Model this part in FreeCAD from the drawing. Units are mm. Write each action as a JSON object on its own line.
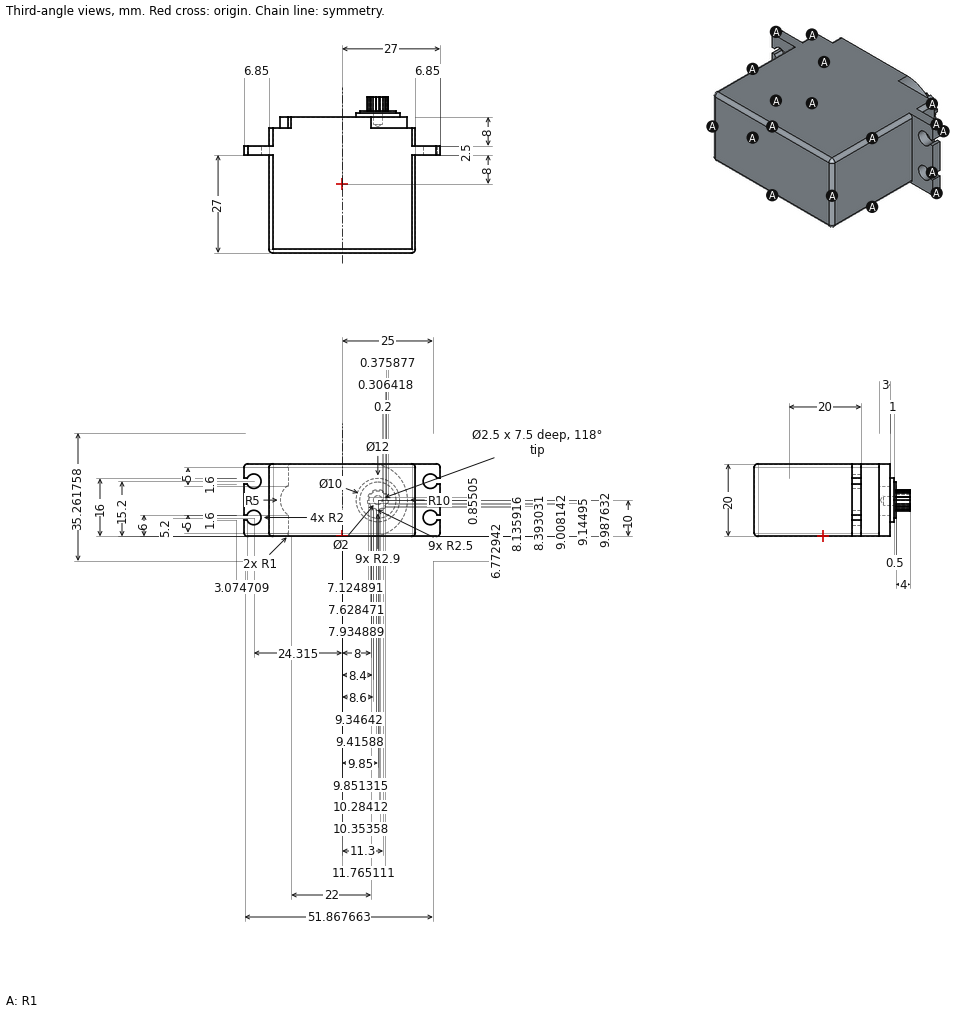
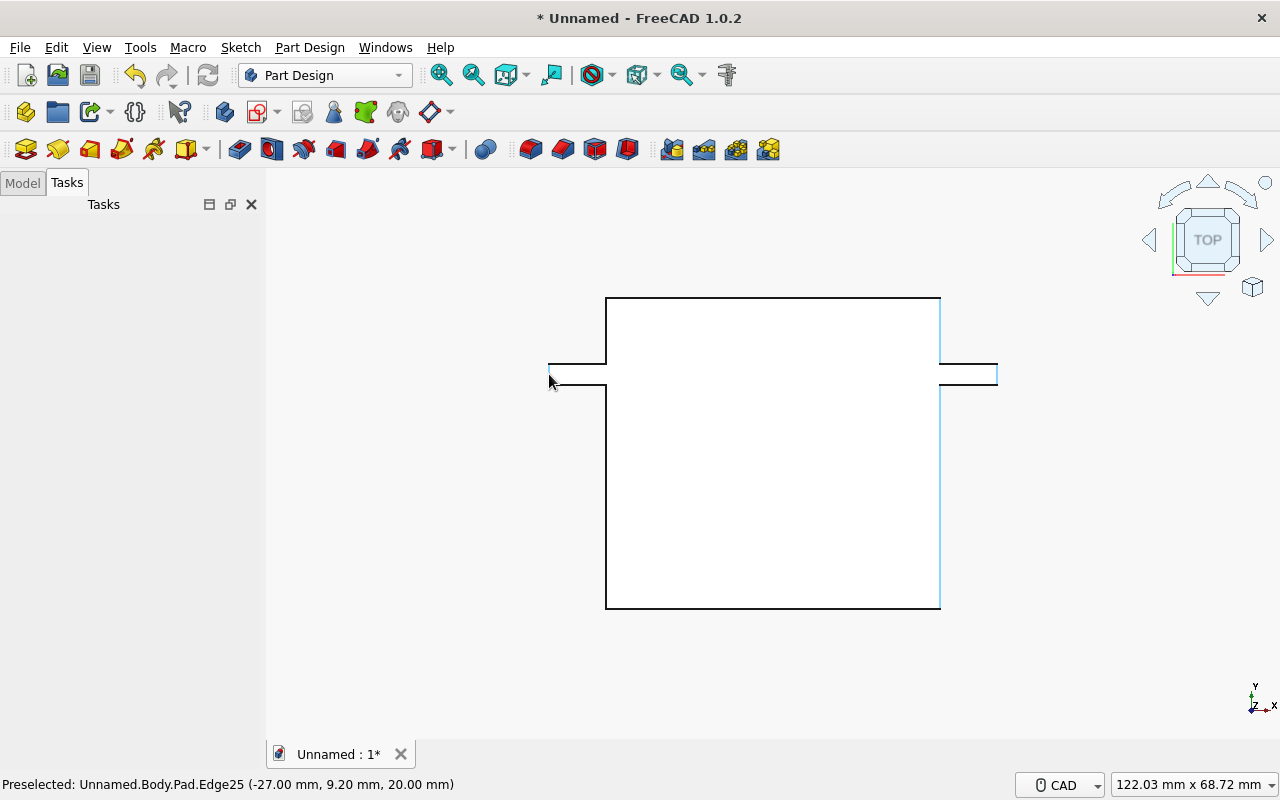
{"action": "left_click", "coordinate": [606, 496], "text": "ctrl"}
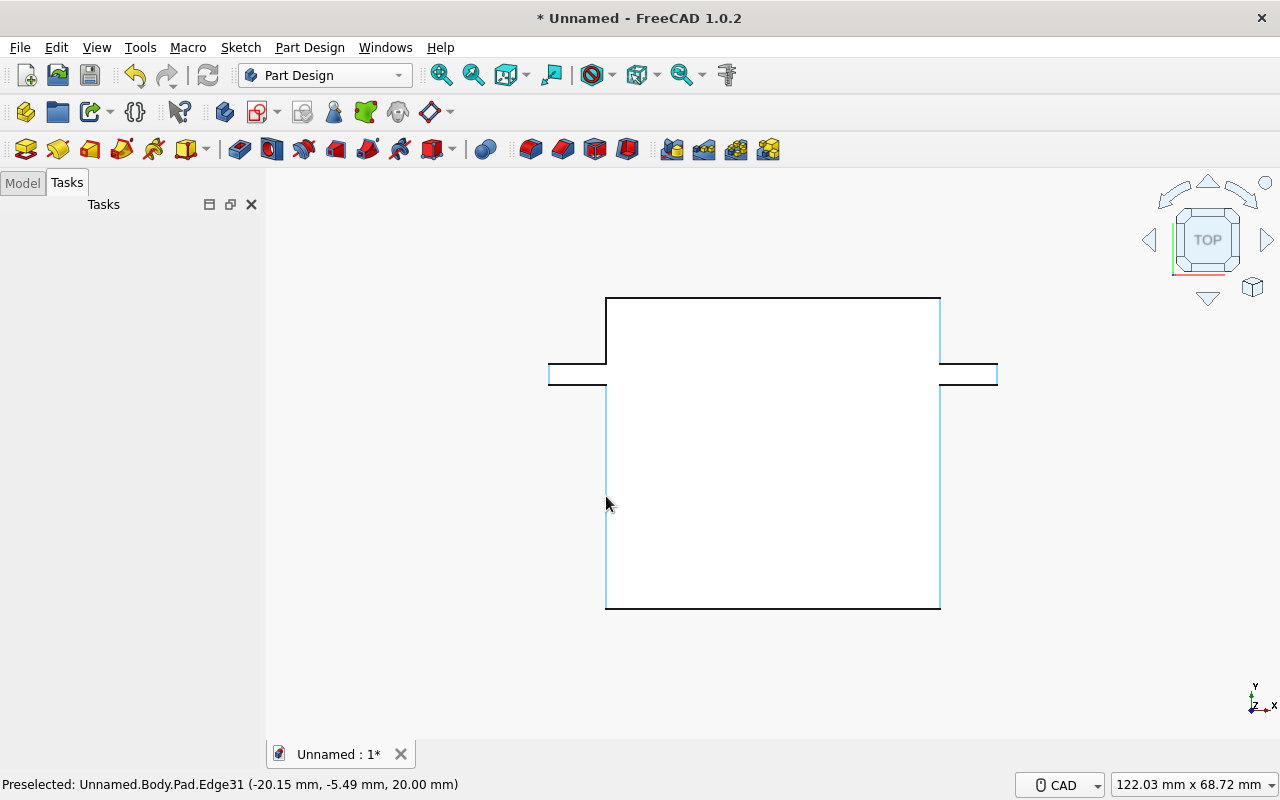
{"action": "left_click", "coordinate": [606, 330], "text": "ctrl"}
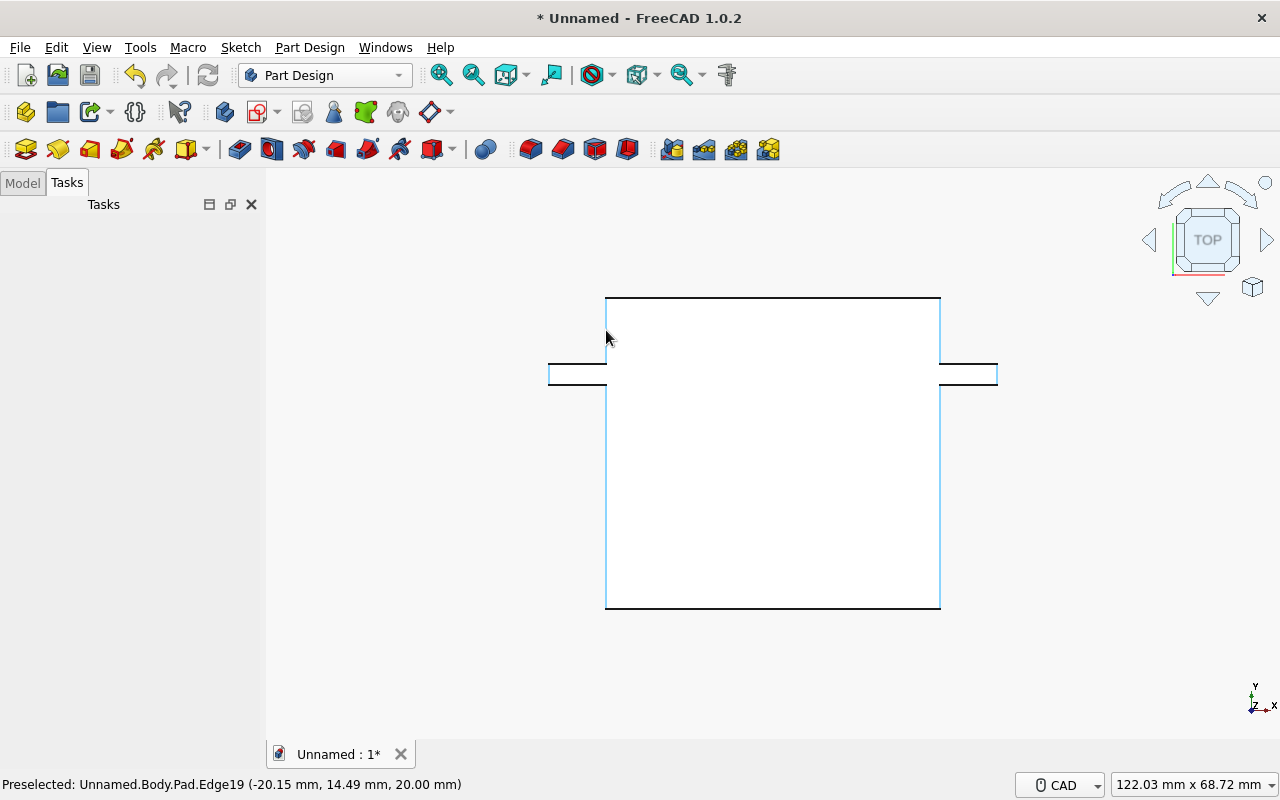
{"action": "key", "text": "1"}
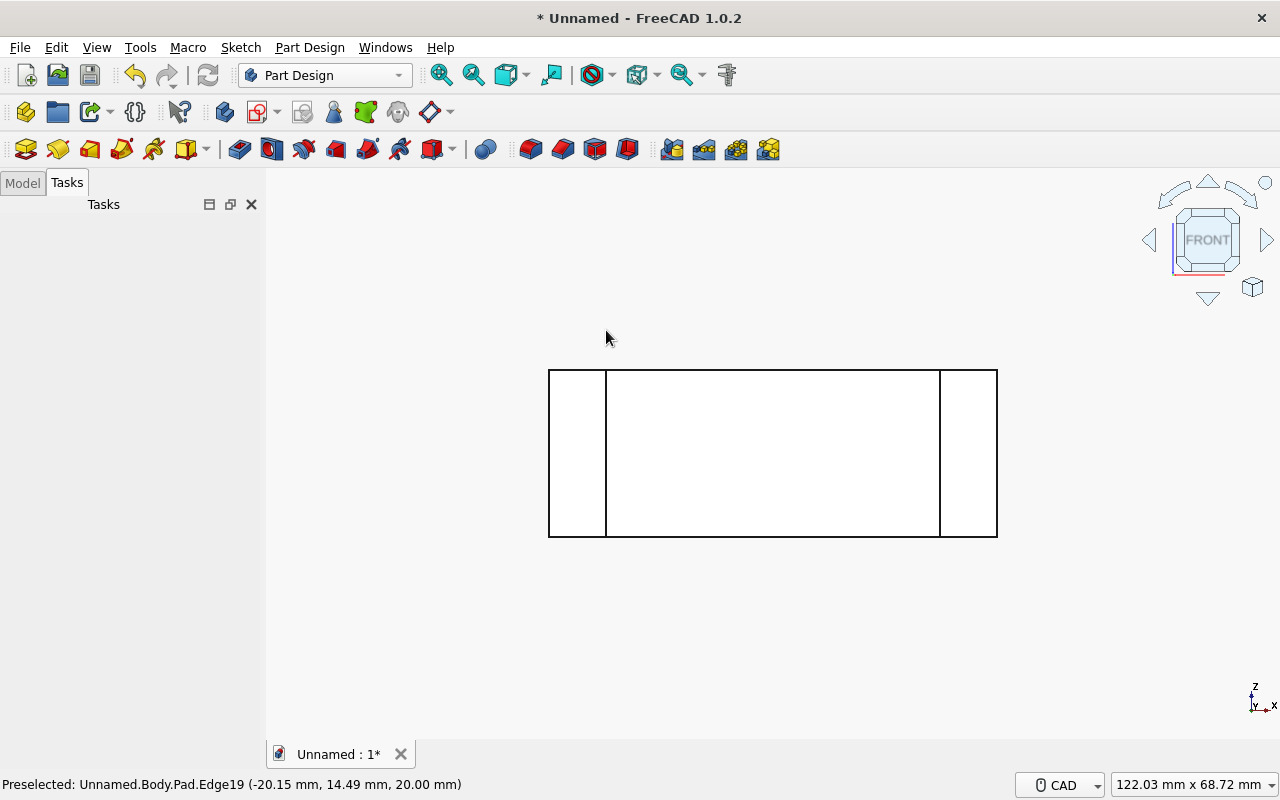
{"action": "key", "text": "v f"}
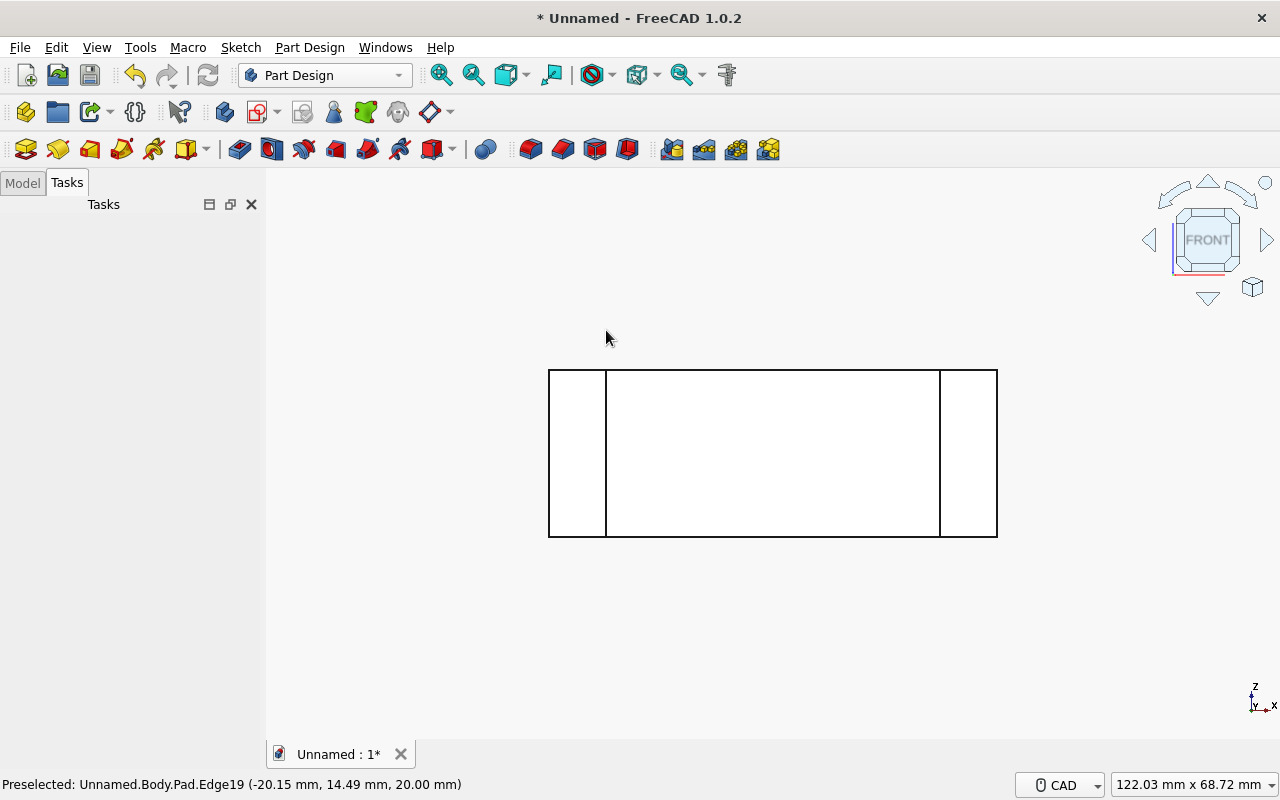
{"action": "key", "text": "3"}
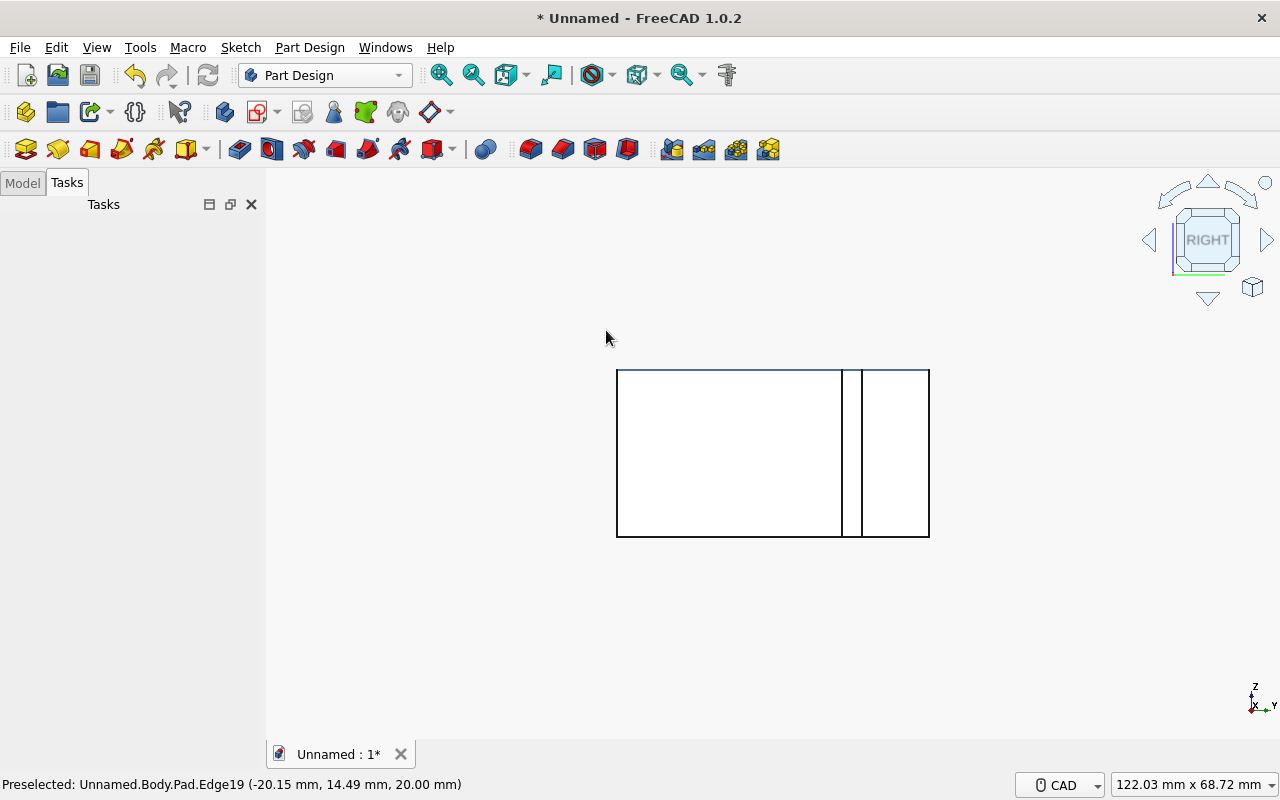
{"action": "key", "text": "v f"}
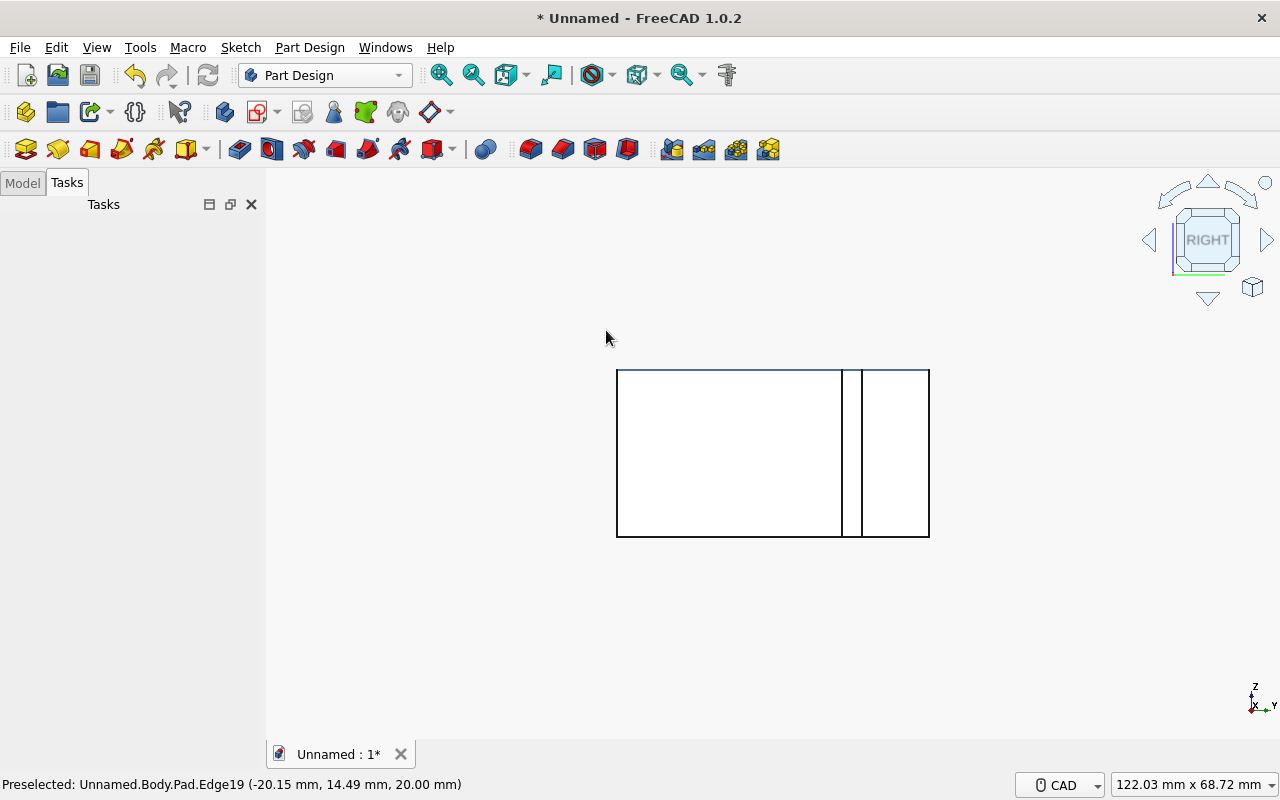
{"action": "left_click", "coordinate": [896, 536], "text": "ctrl"}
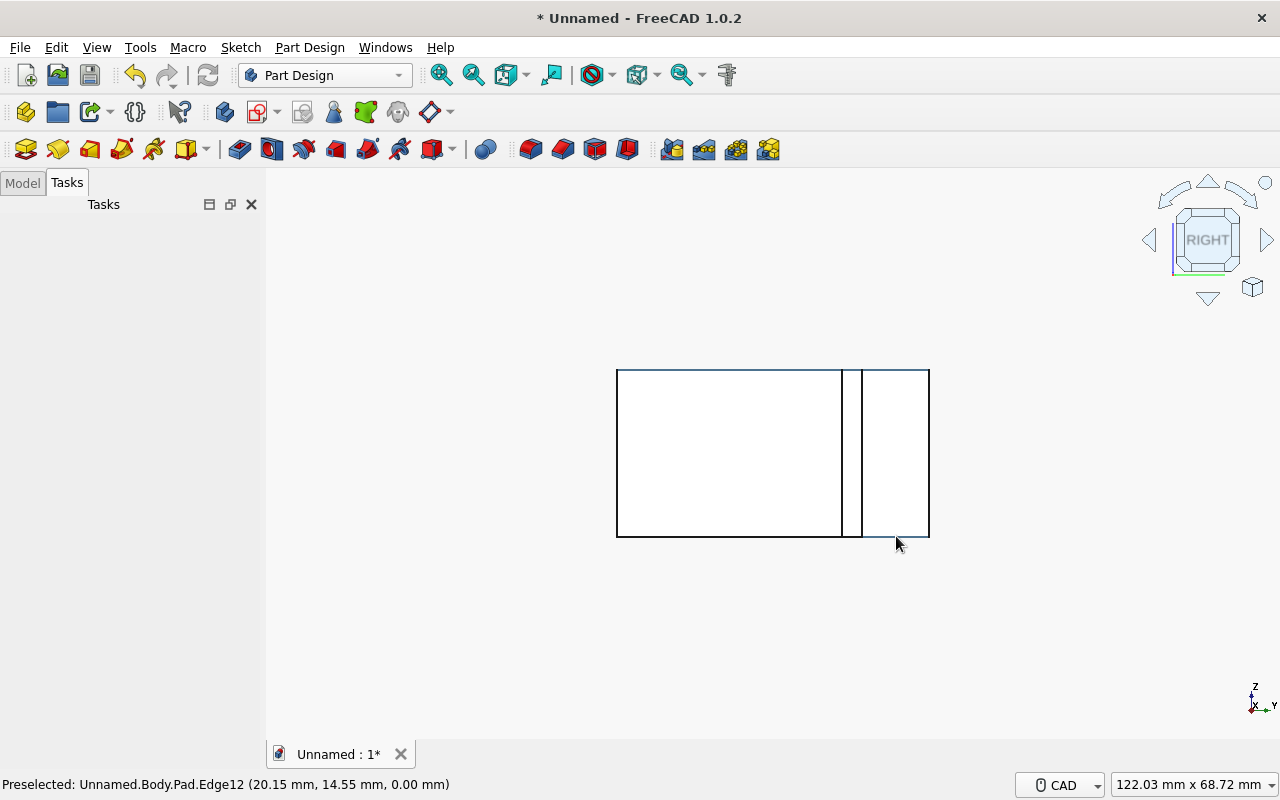
{"action": "left_click", "coordinate": [852, 536], "text": "ctrl"}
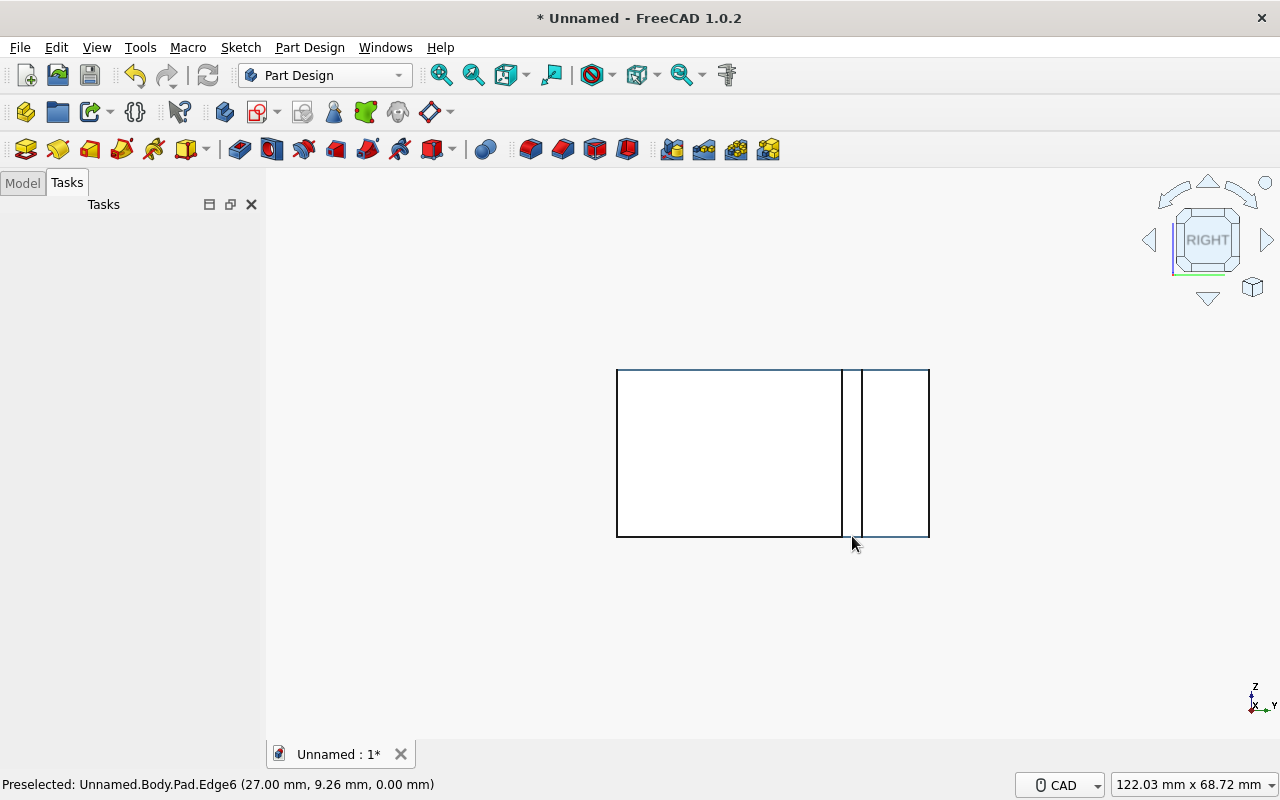
{"action": "left_click", "coordinate": [729, 536], "text": "ctrl"}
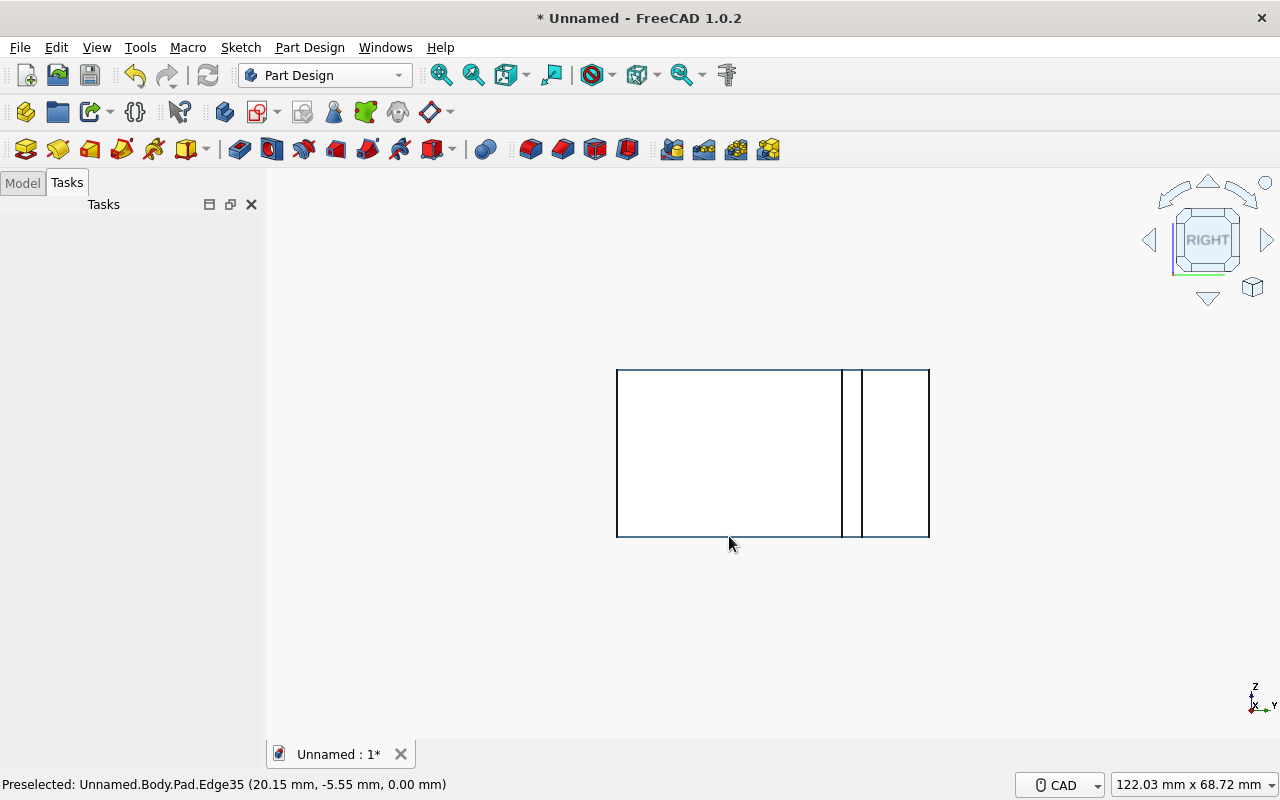
{"action": "left_click", "coordinate": [929, 452], "text": "ctrl"}